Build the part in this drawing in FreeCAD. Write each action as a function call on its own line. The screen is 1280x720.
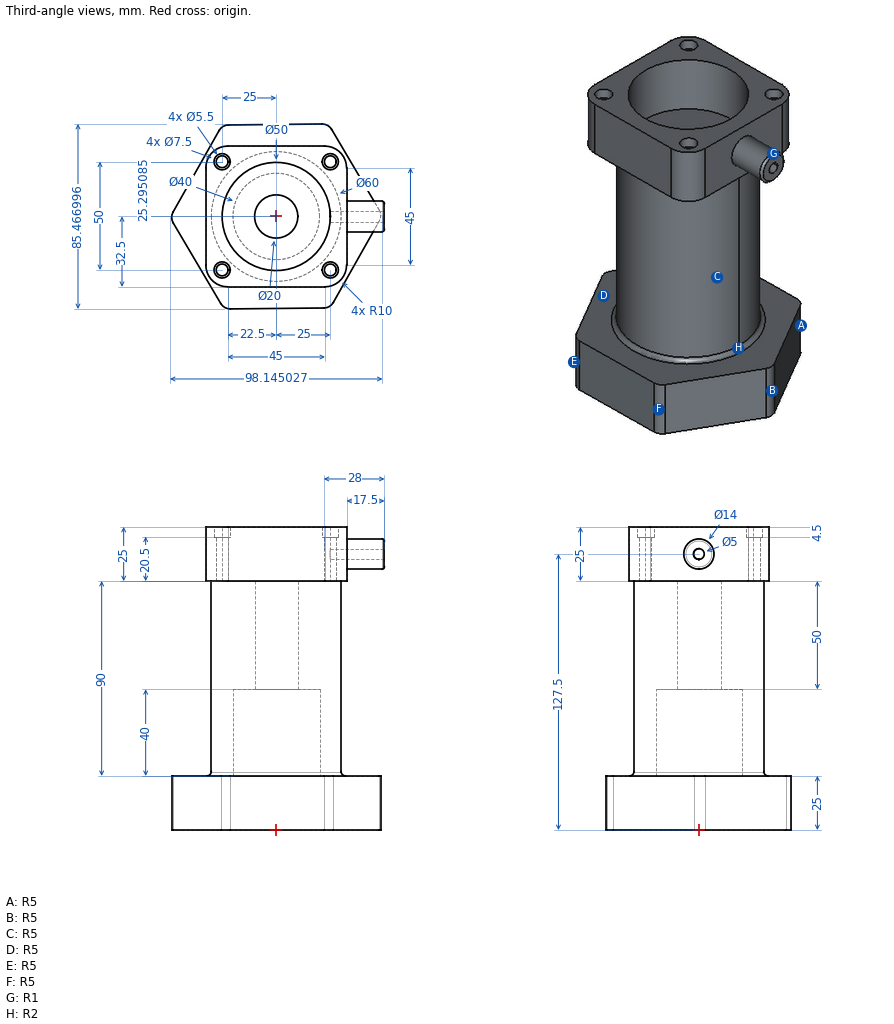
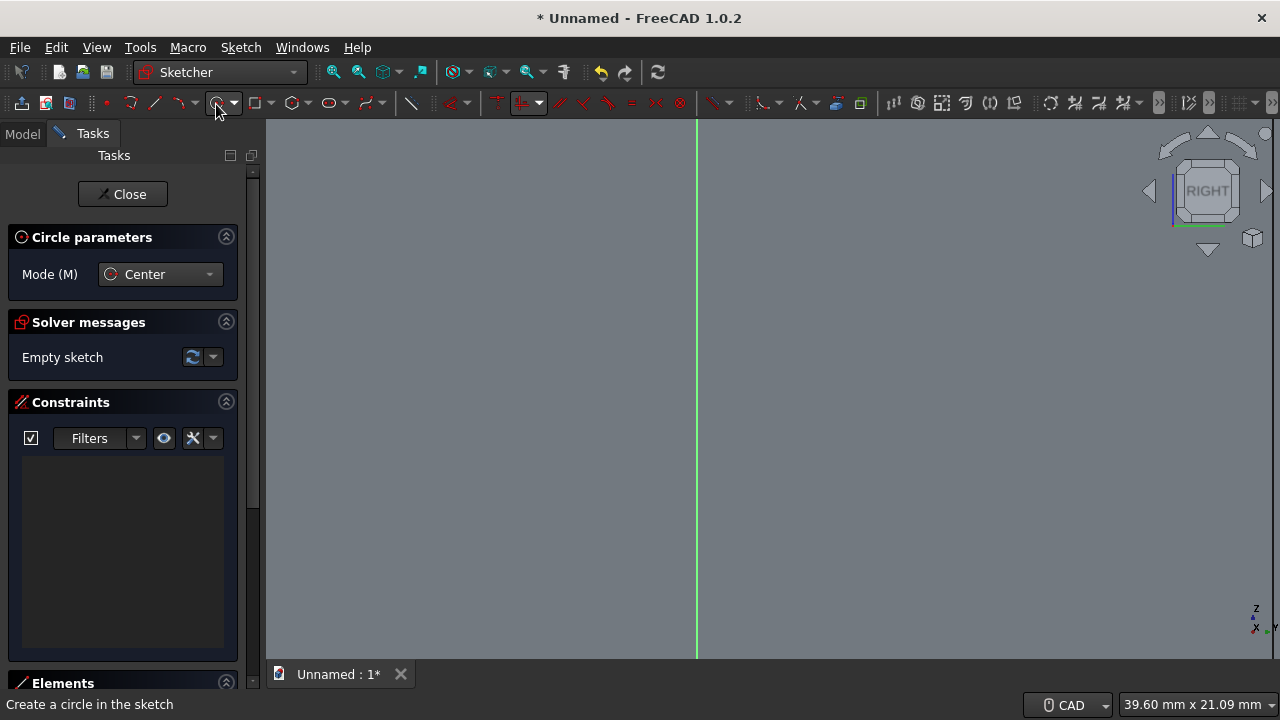
click(697, 384)
click(824, 257)
key(Escape)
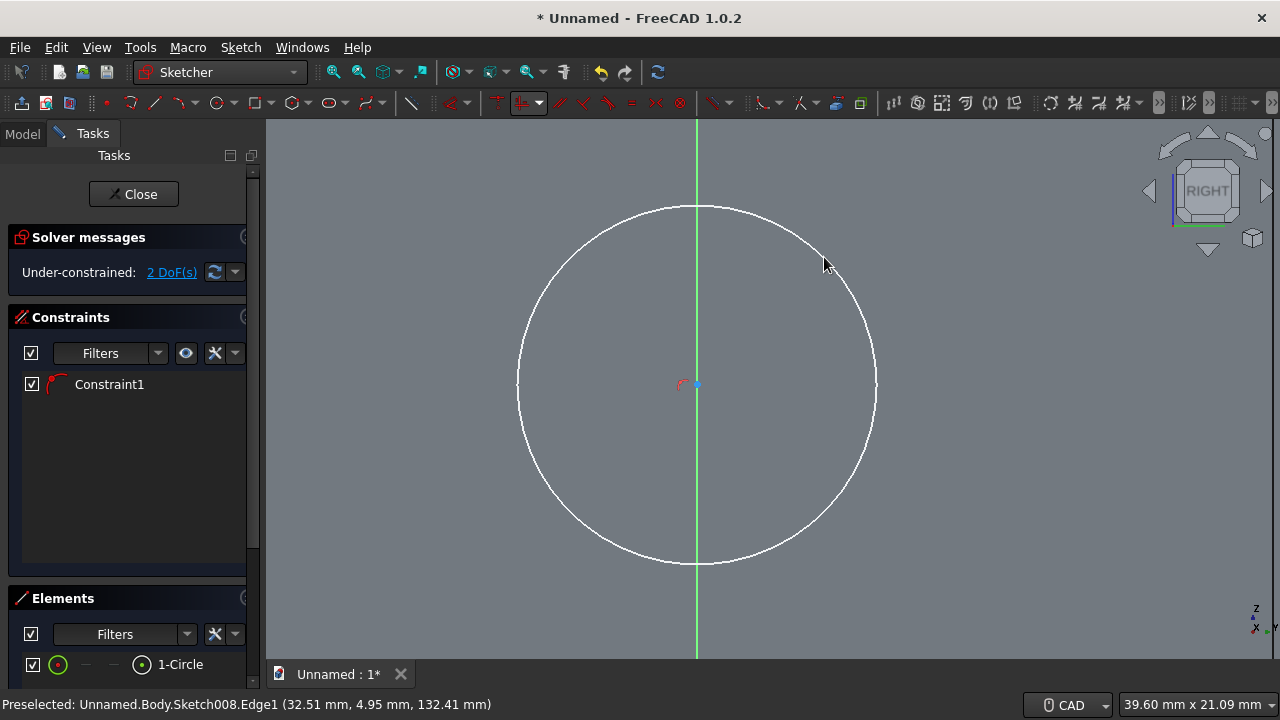
click(450, 104)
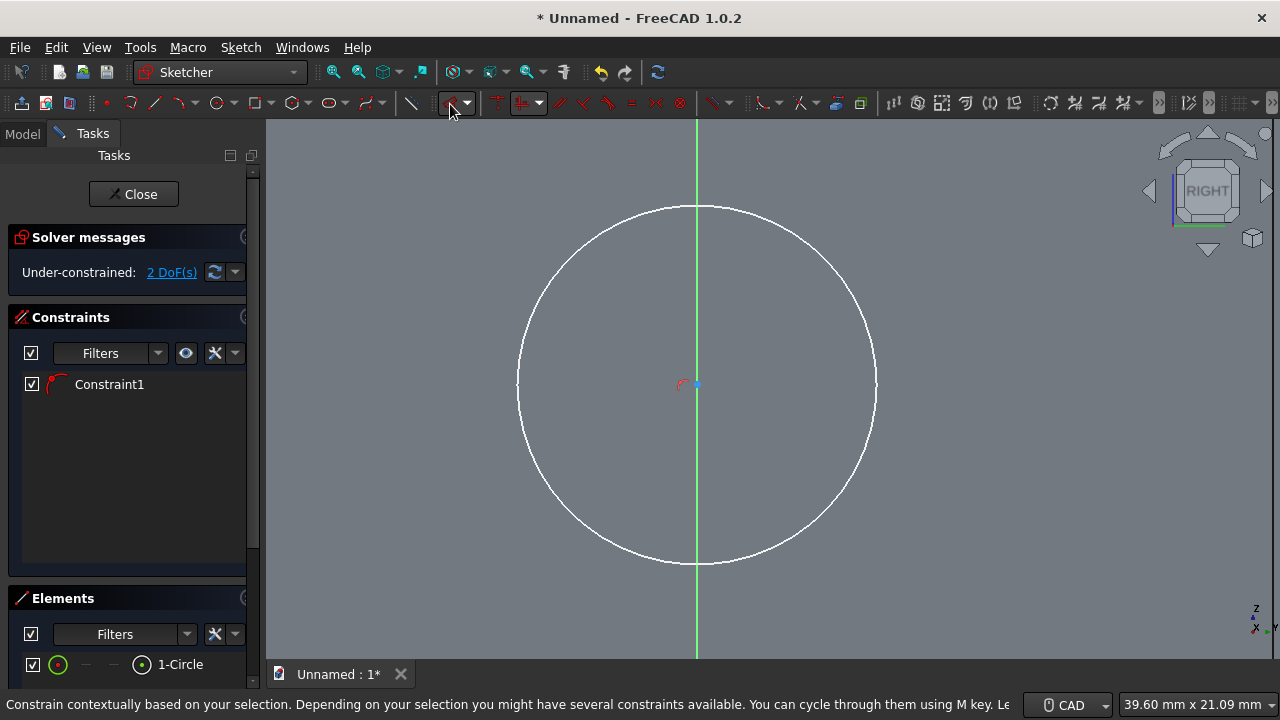
click(824, 258)
click(847, 235)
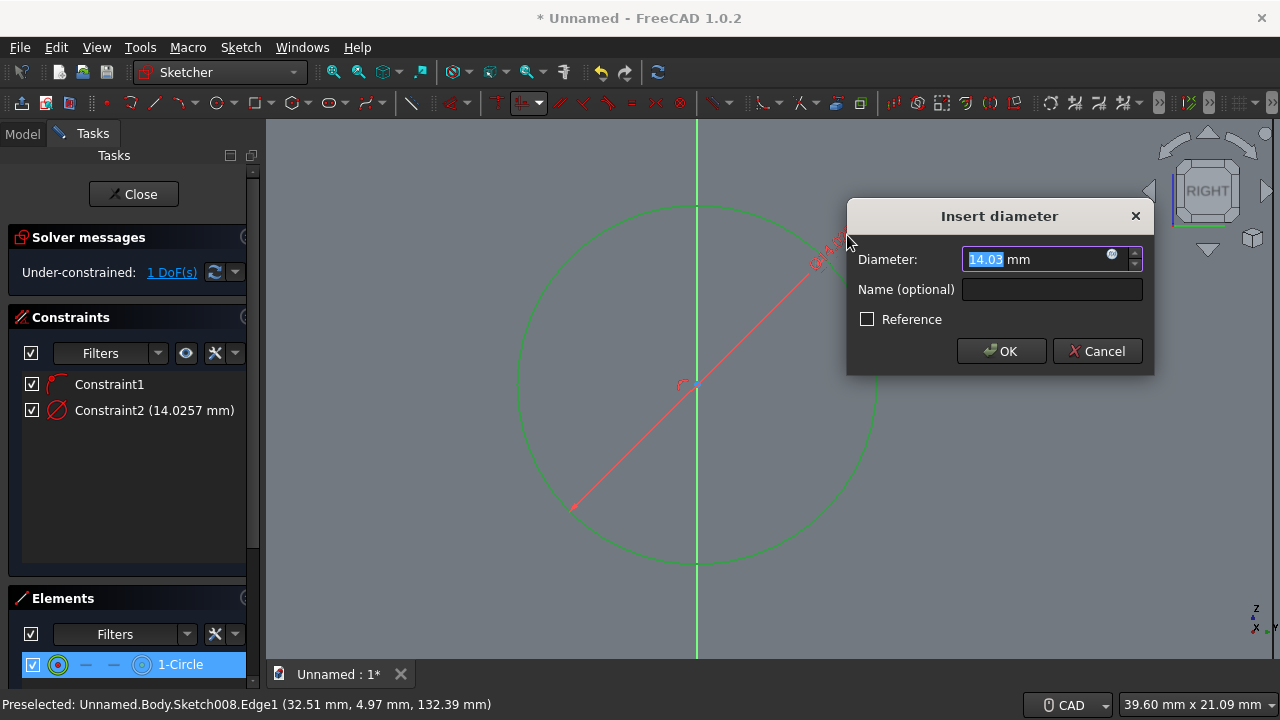
text(14)
key(Return)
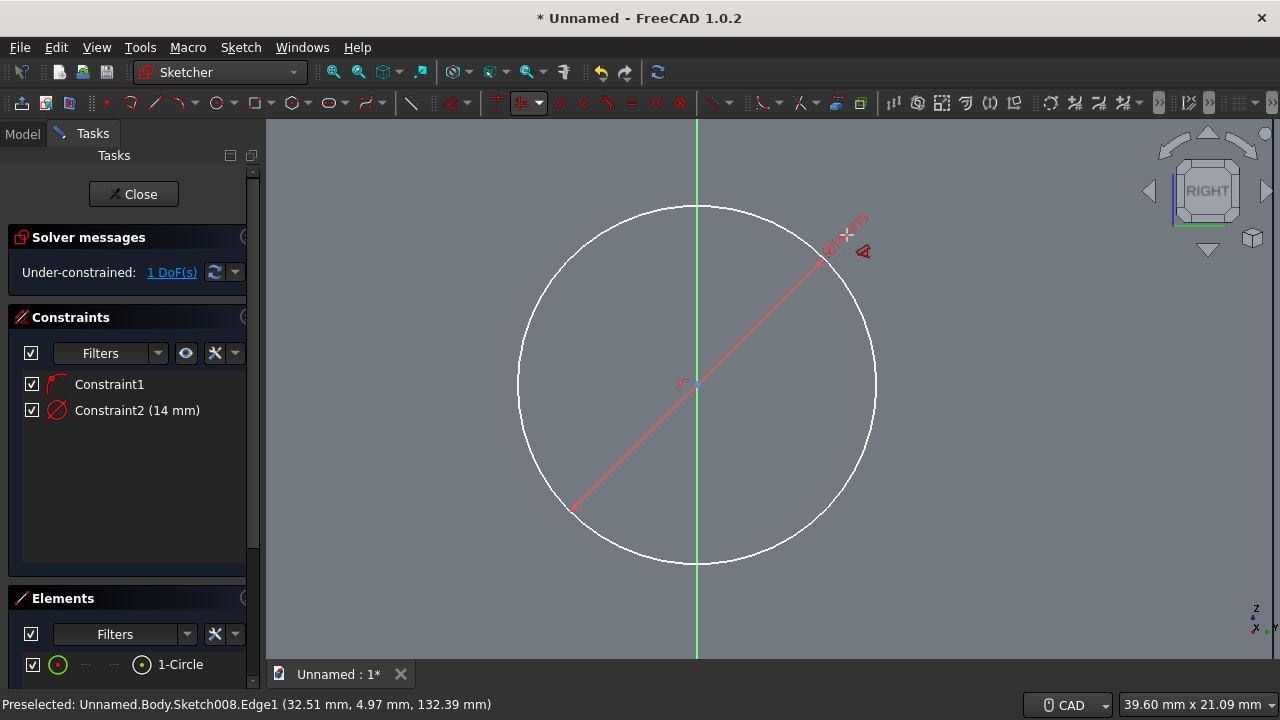
click(697, 385)
click(731, 508)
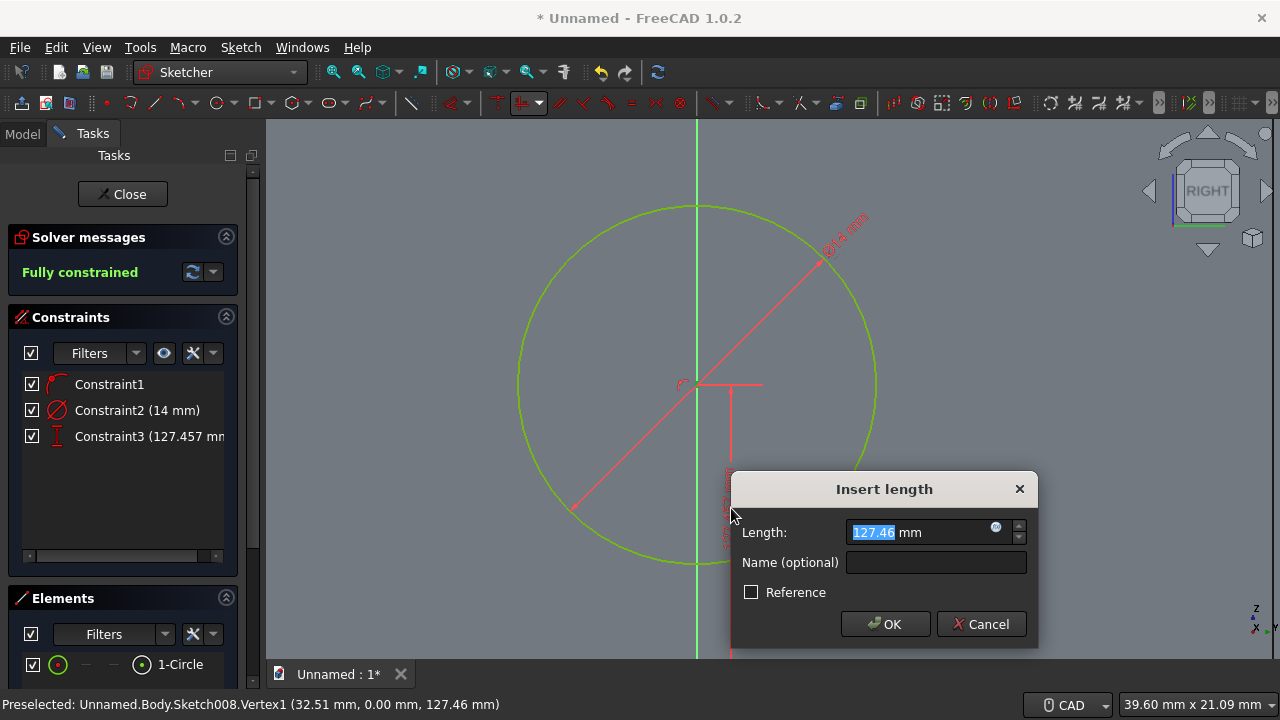
text(127.5)
key(Return)
key(Escape)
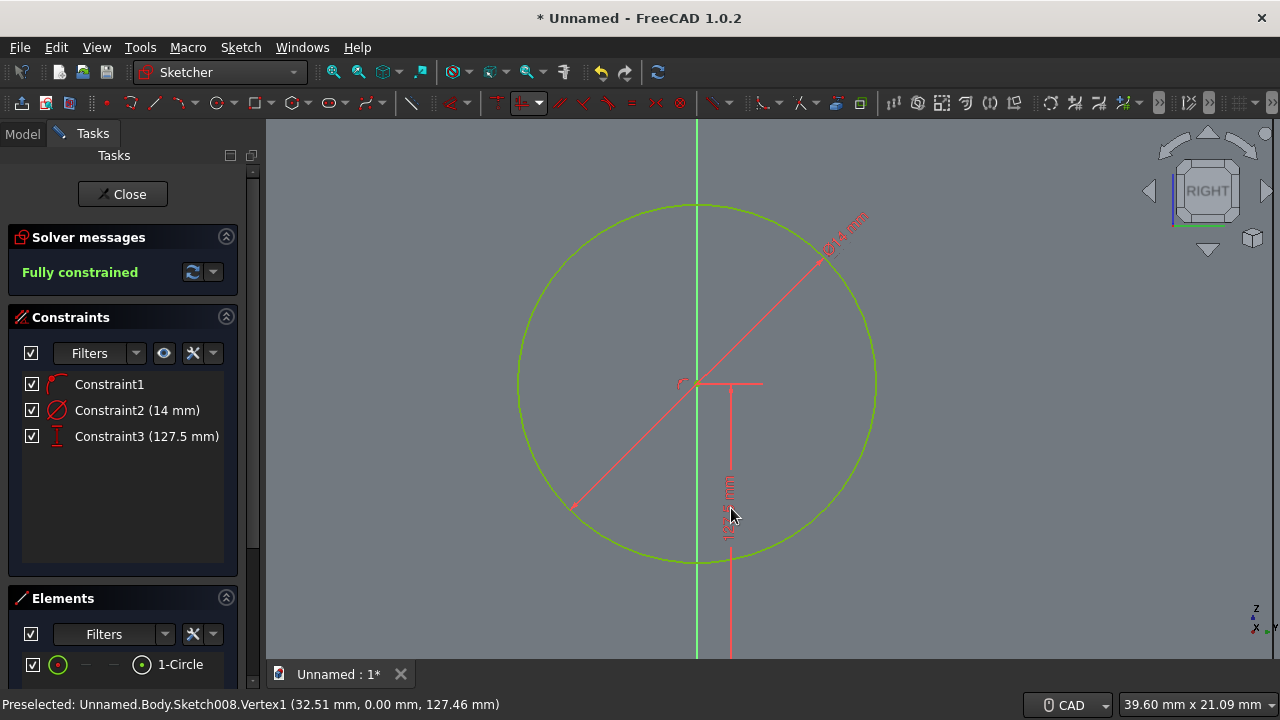
click(123, 194)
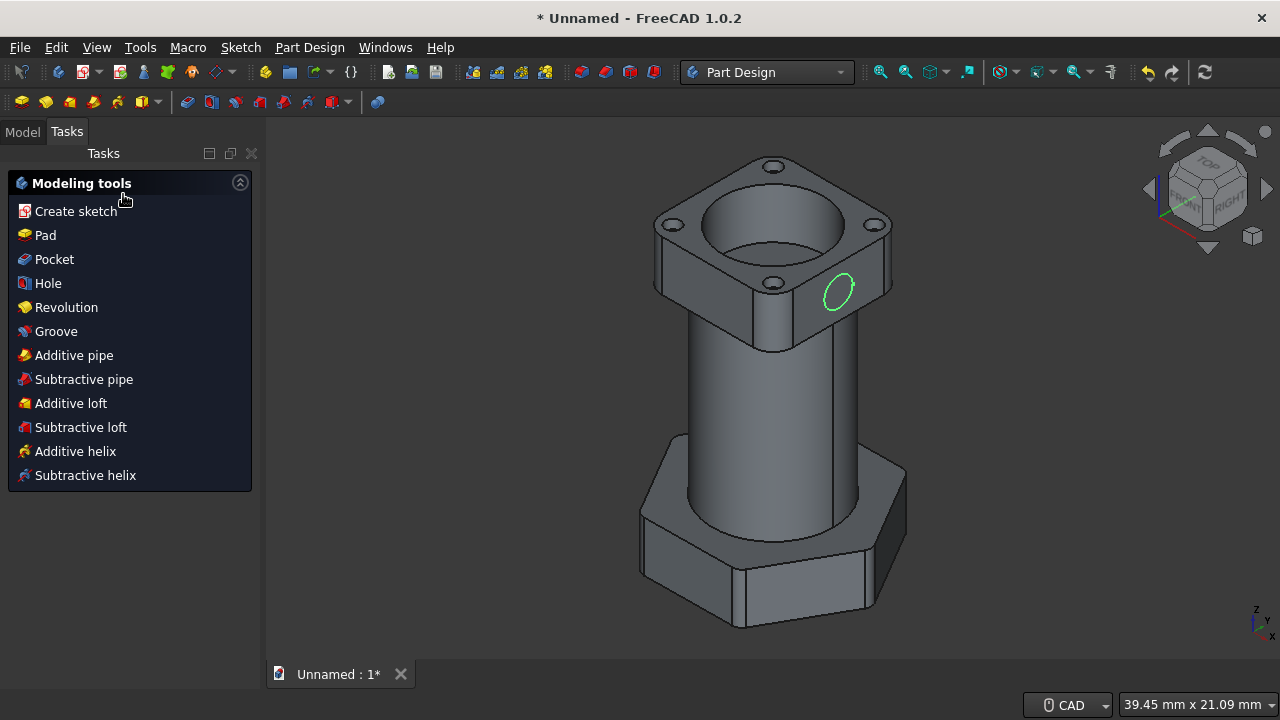
click(22, 102)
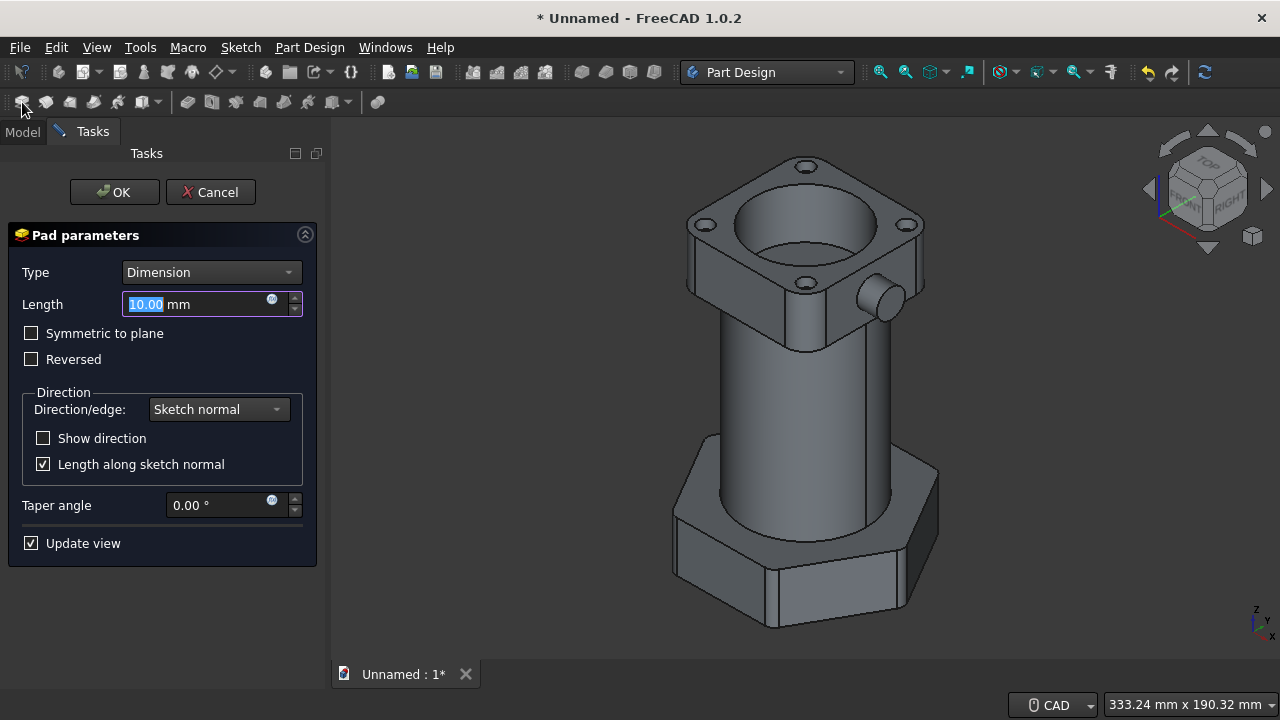
text(17.5)
key(Tab)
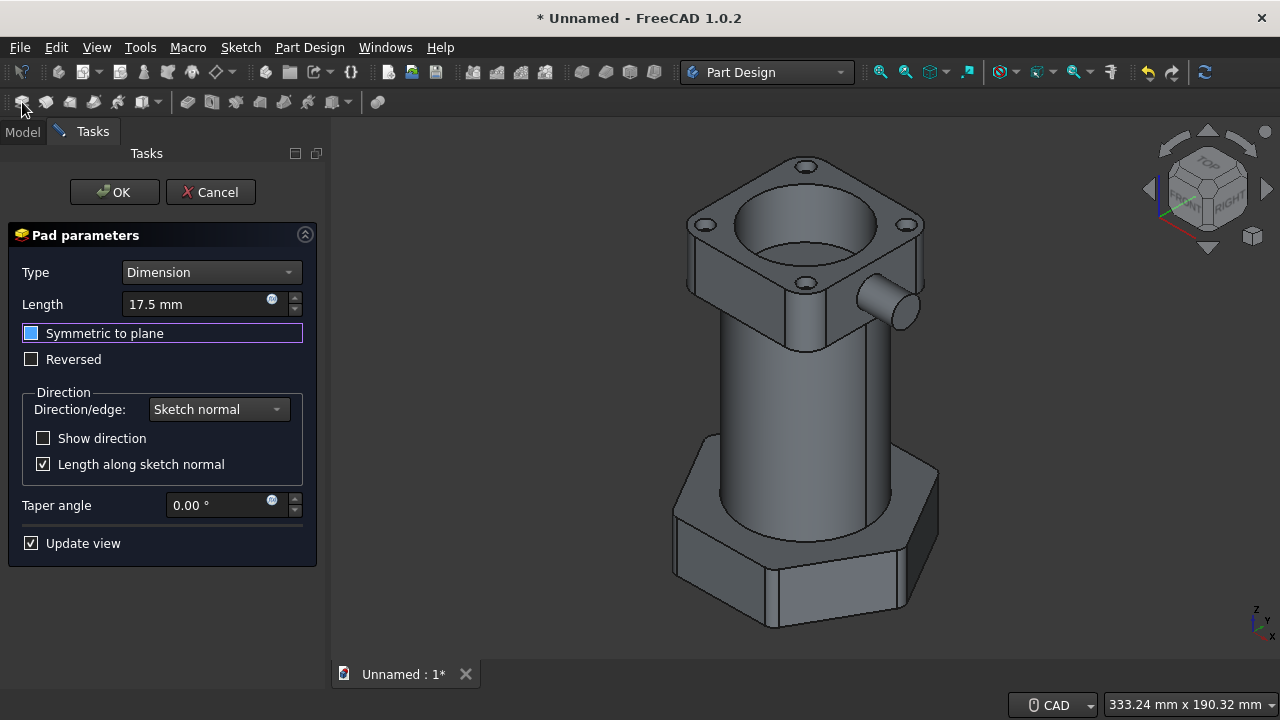
click(115, 192)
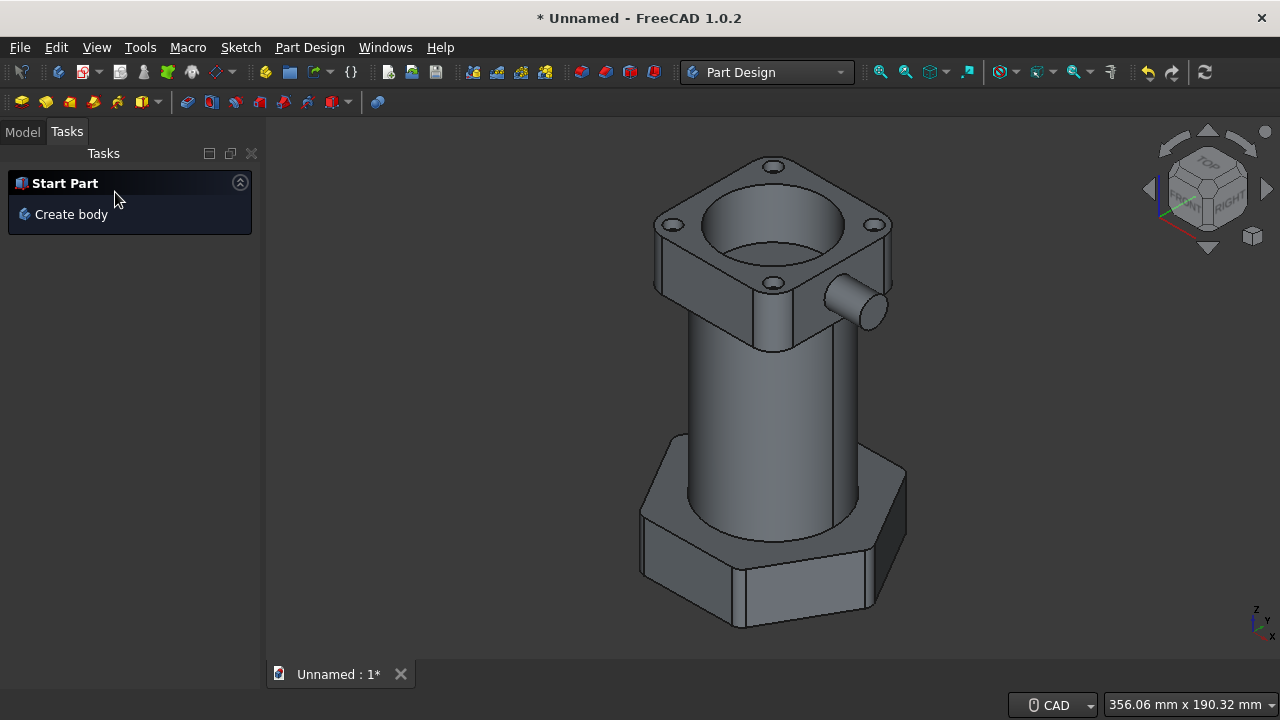
click(860, 320)